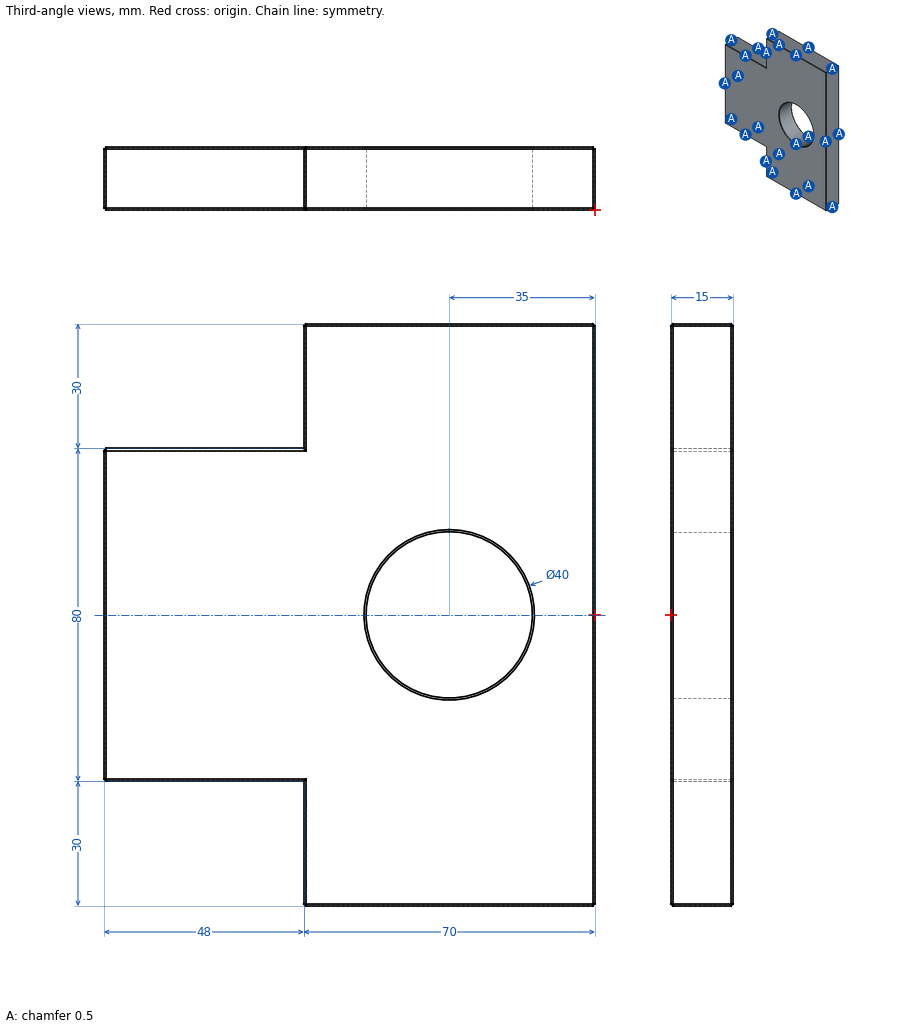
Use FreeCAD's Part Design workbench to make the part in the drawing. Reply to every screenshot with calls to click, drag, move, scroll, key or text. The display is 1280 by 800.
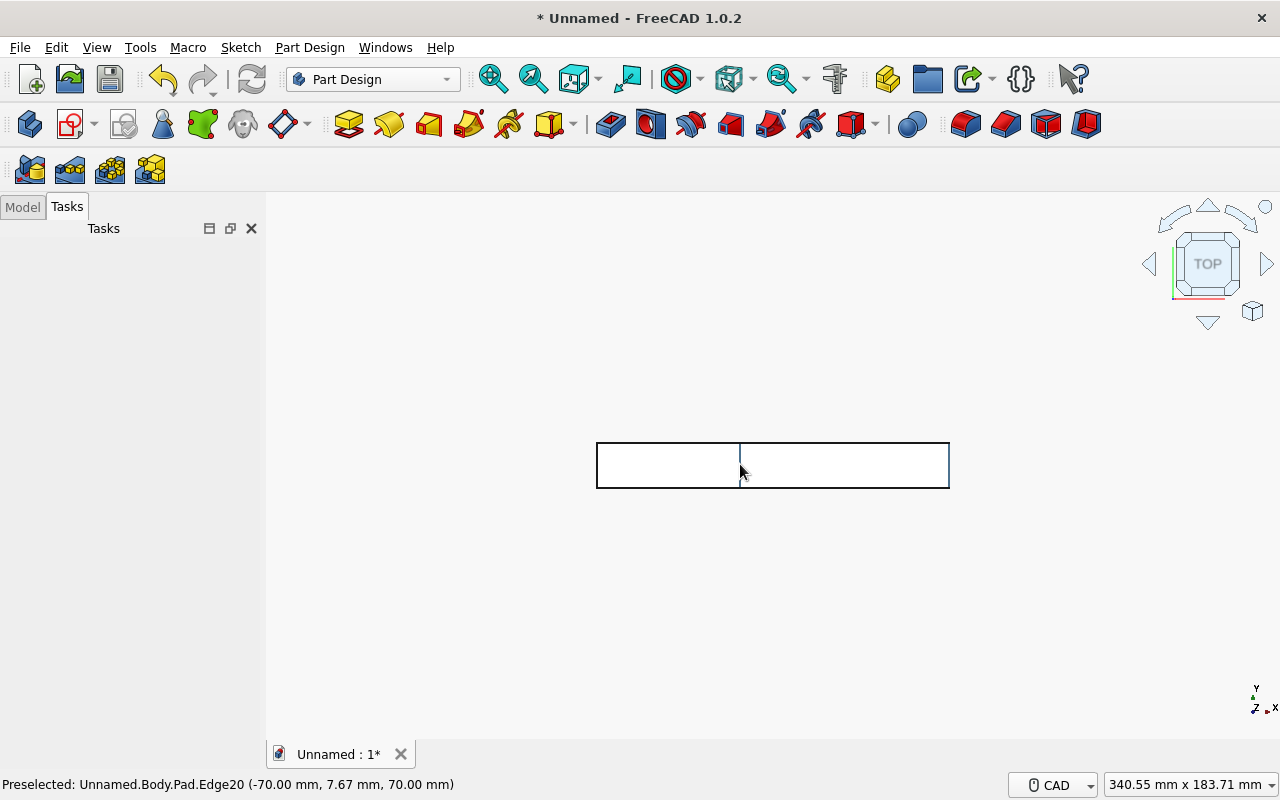
click(597, 464, ctrl)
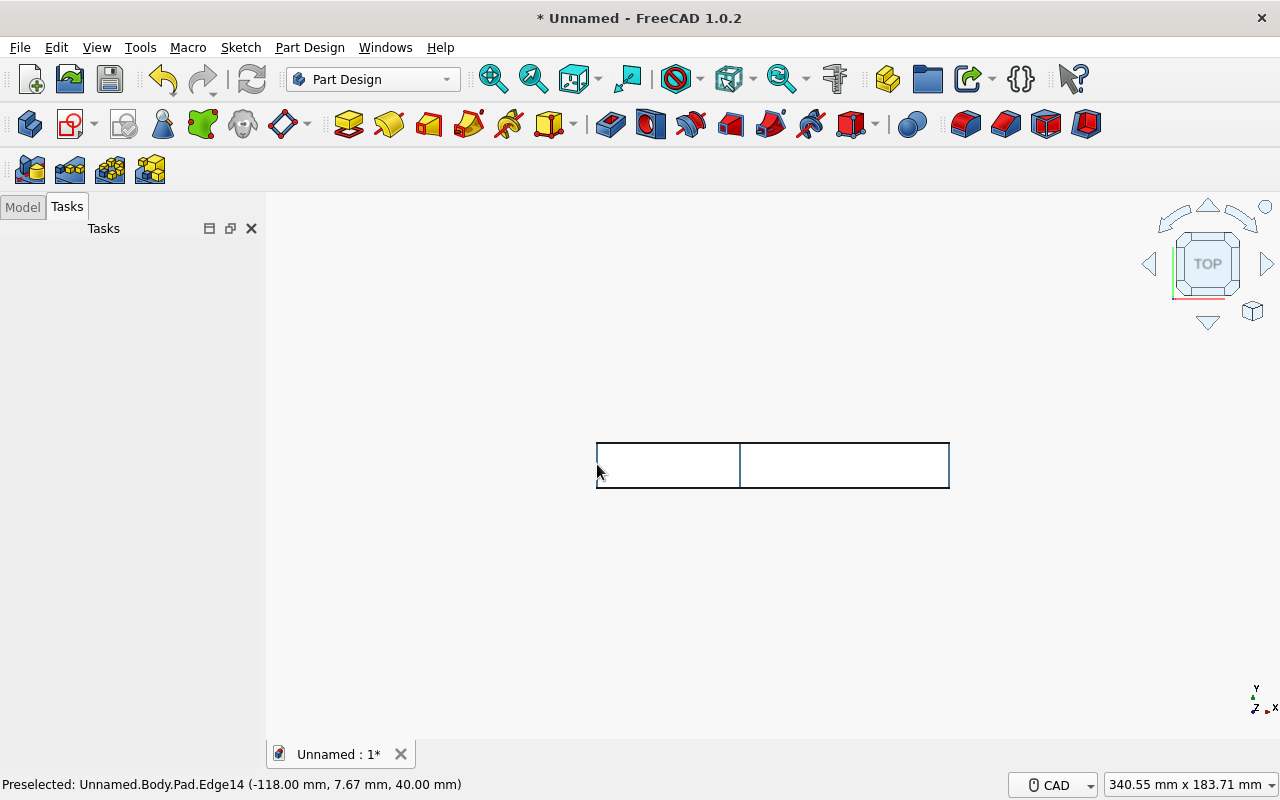
key(1)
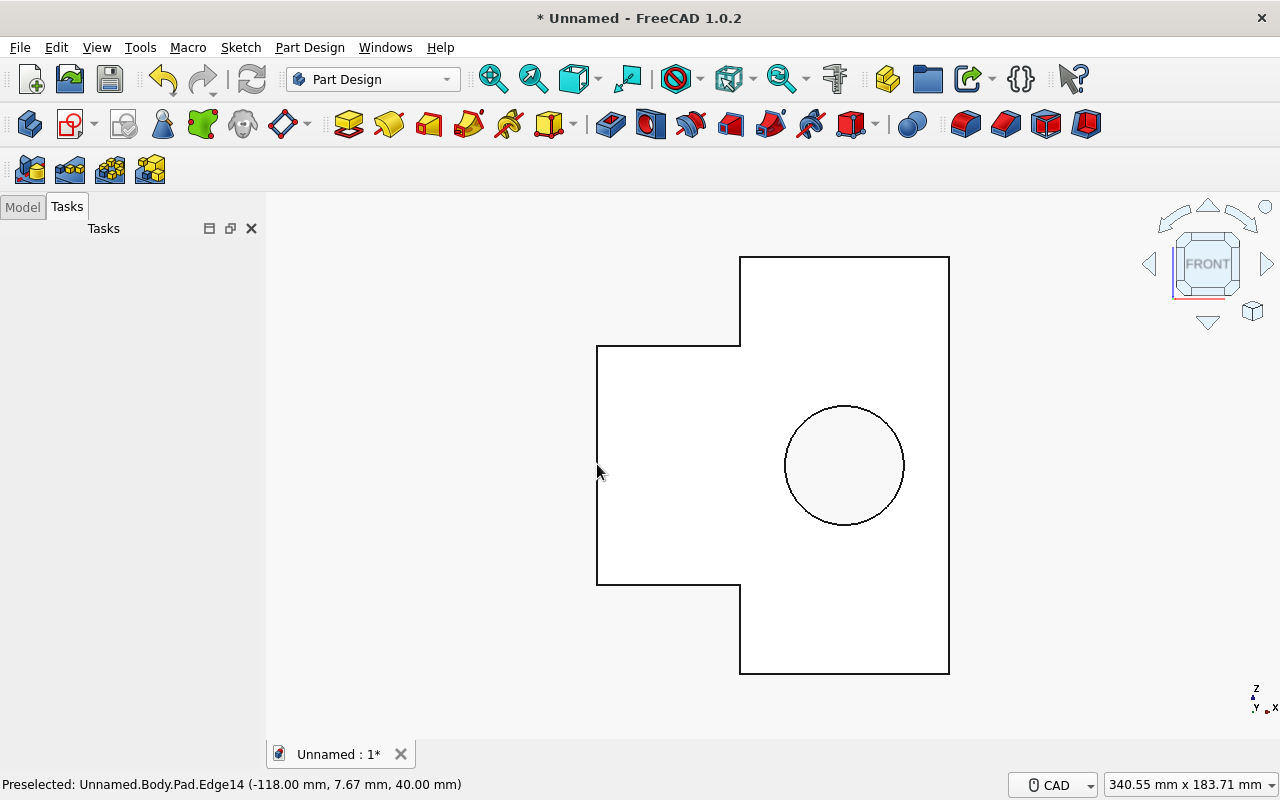
key(3)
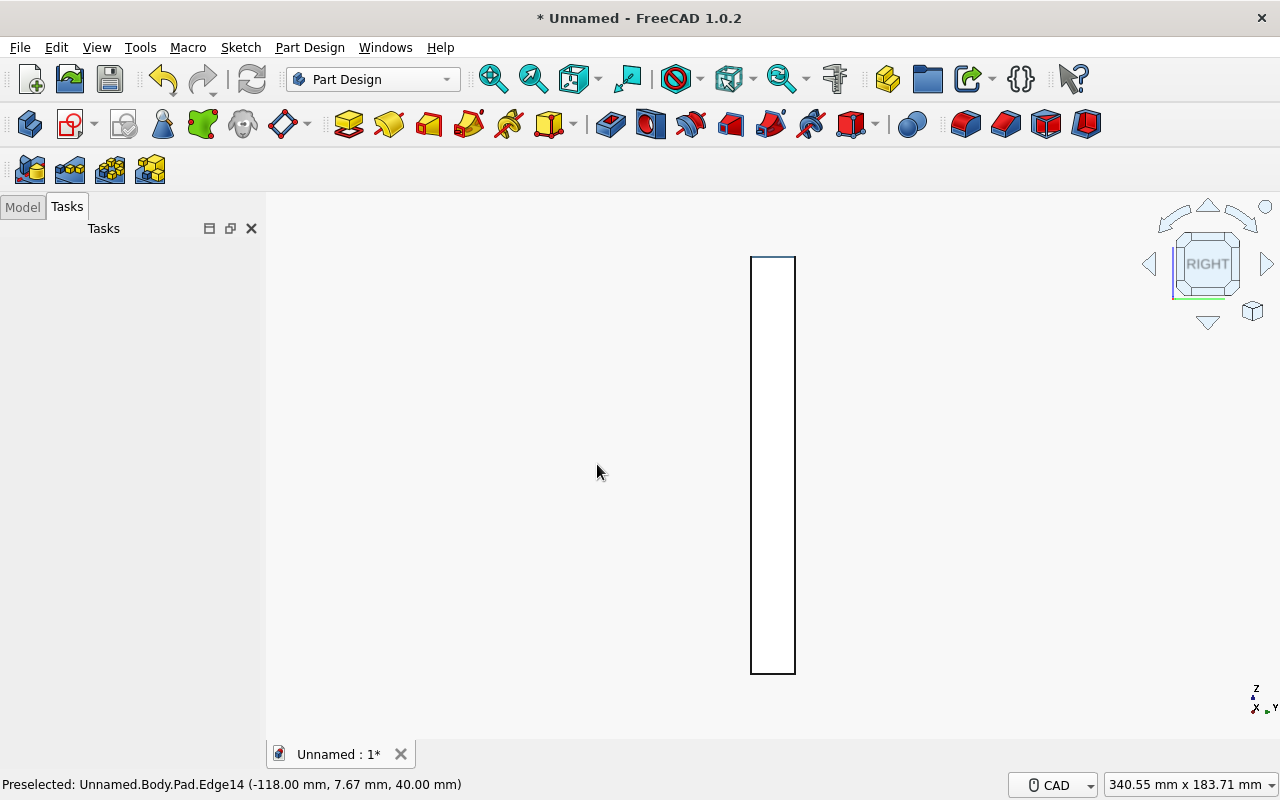
click(773, 673, ctrl)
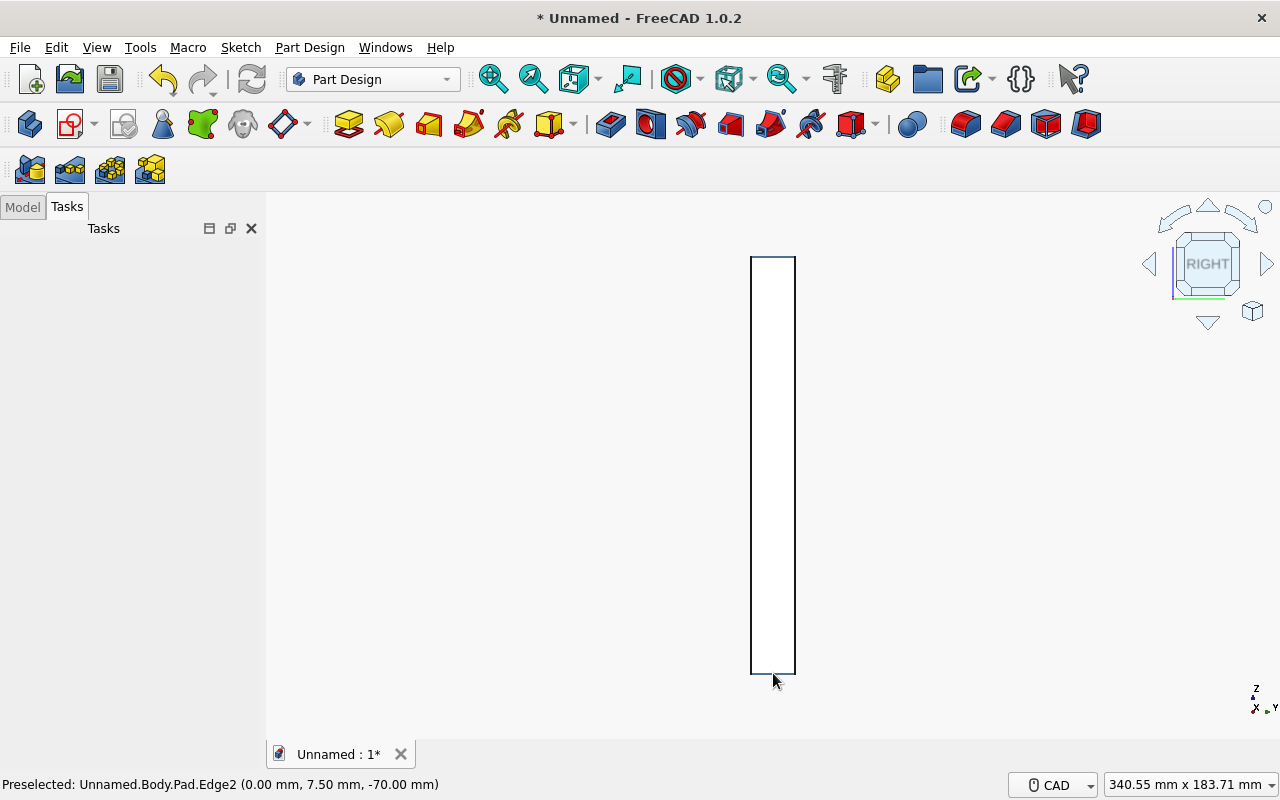
key(5)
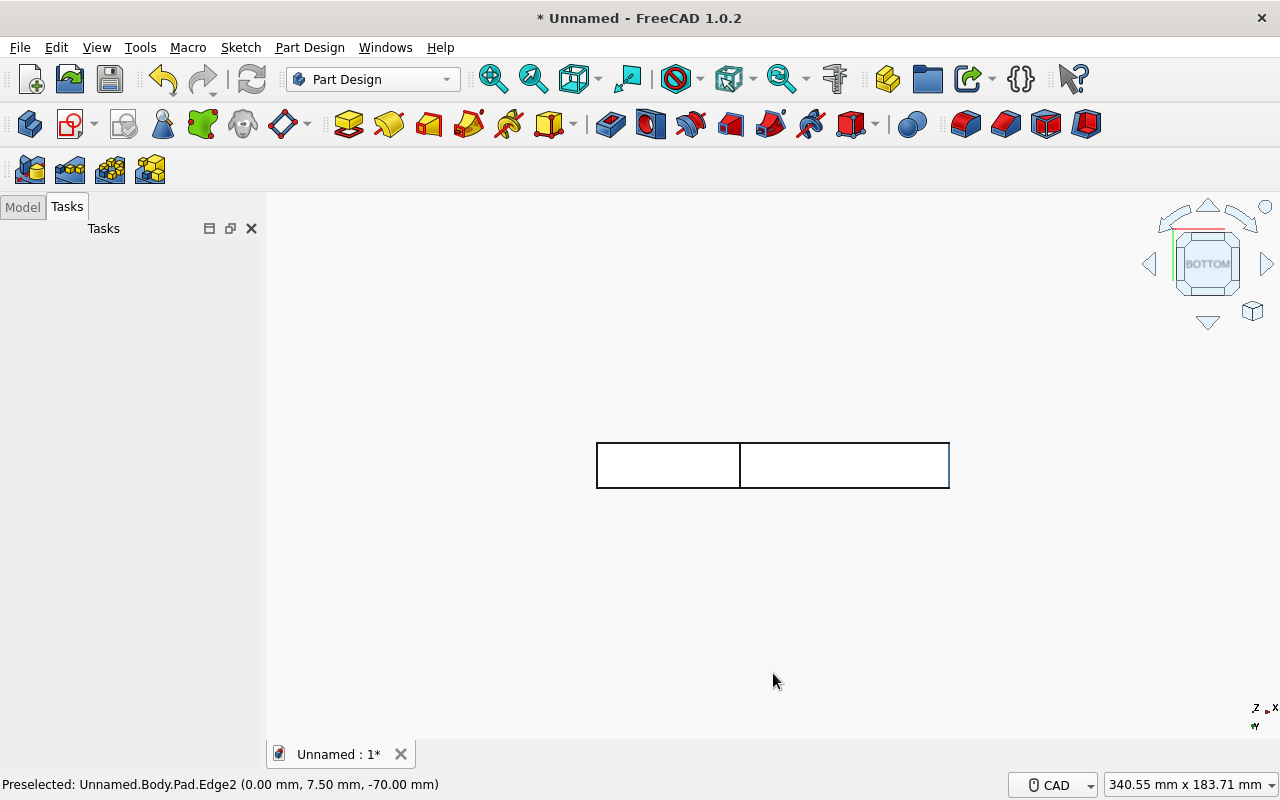
click(494, 80)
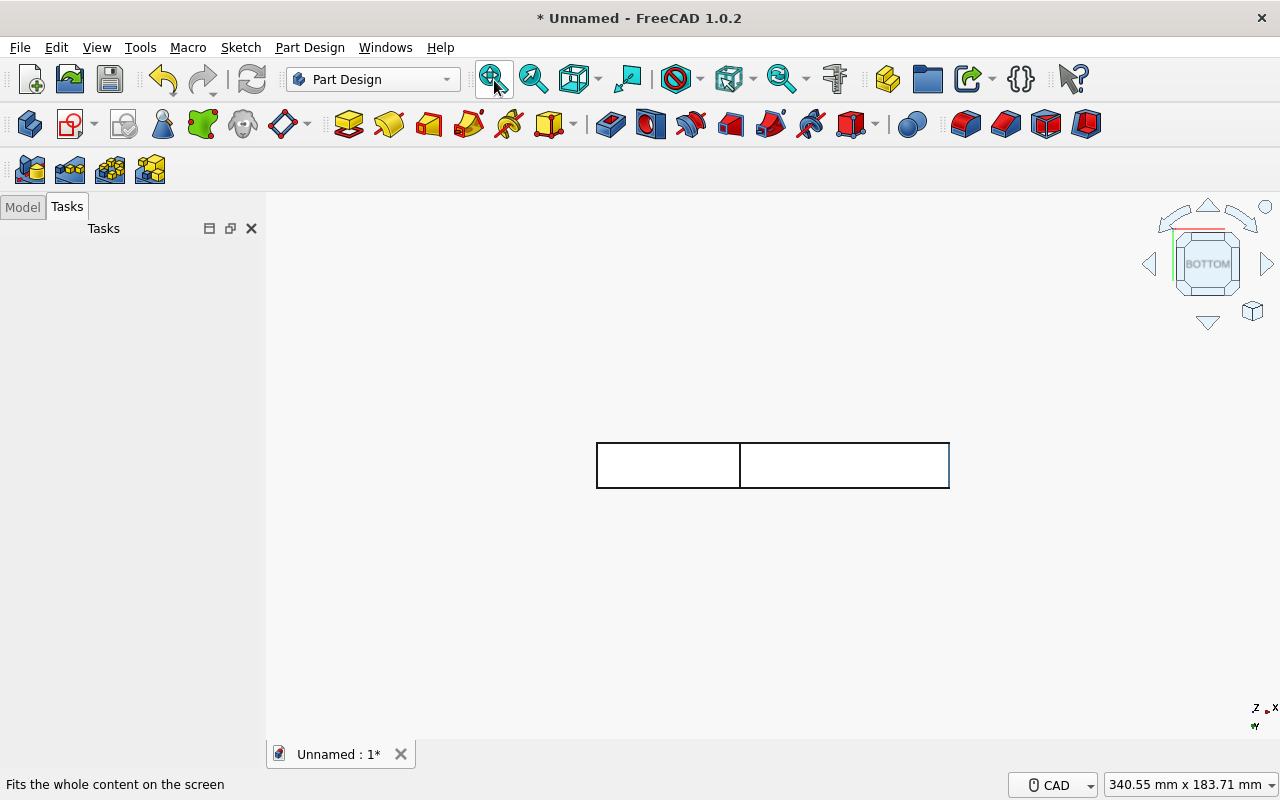
click(597, 464, ctrl)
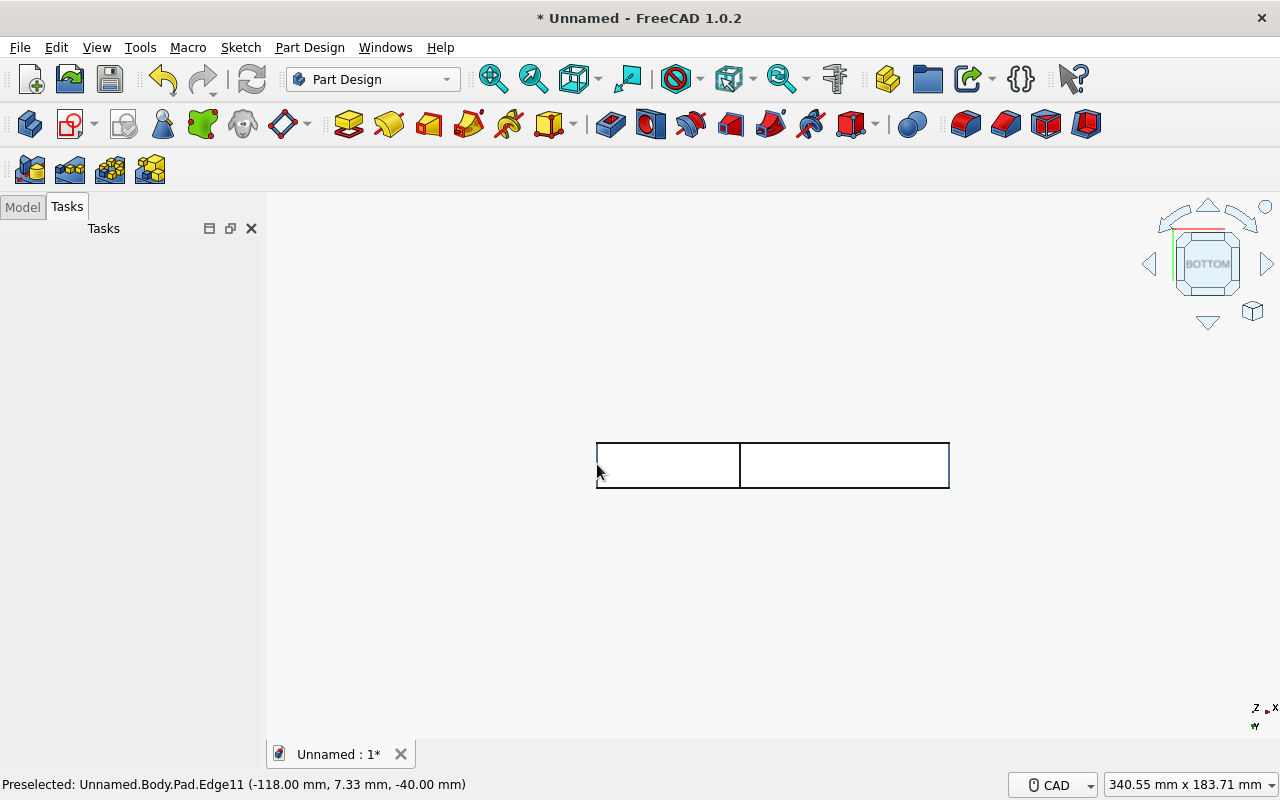
click(740, 464, ctrl)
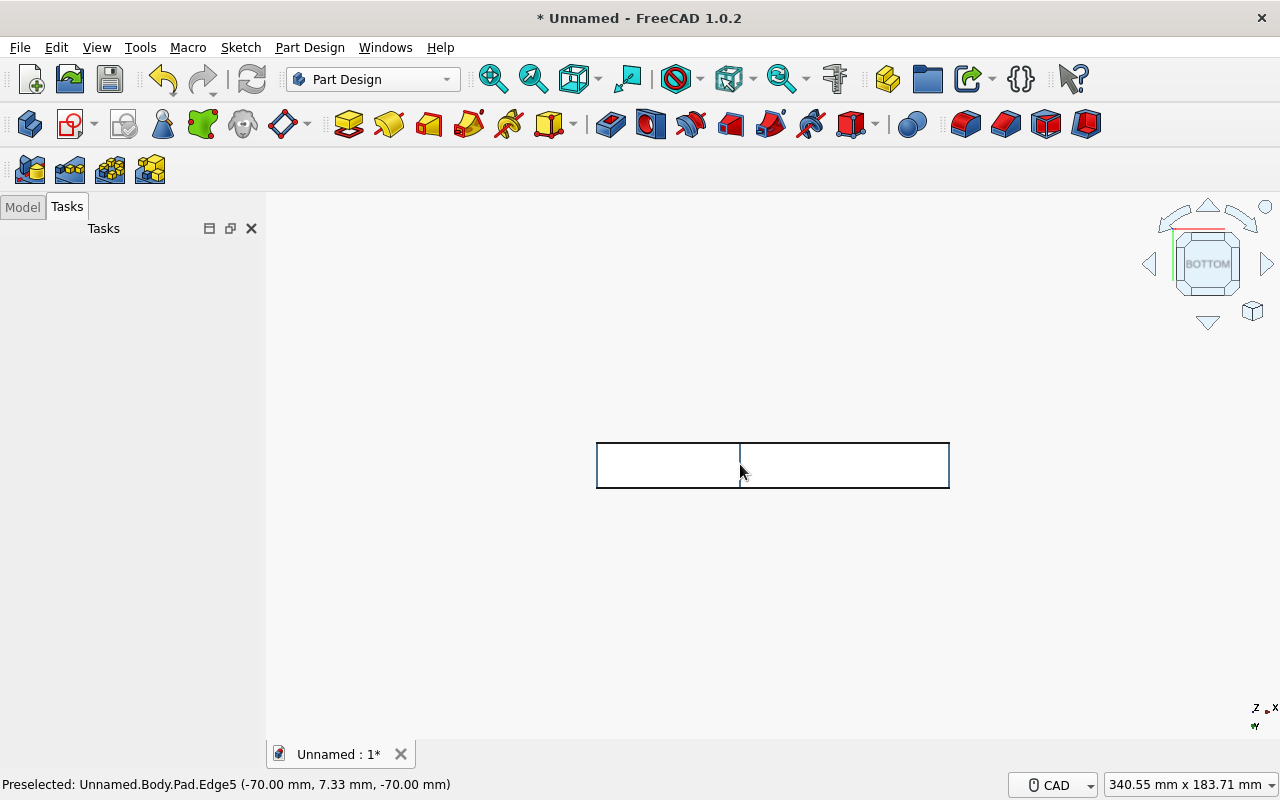
key(4)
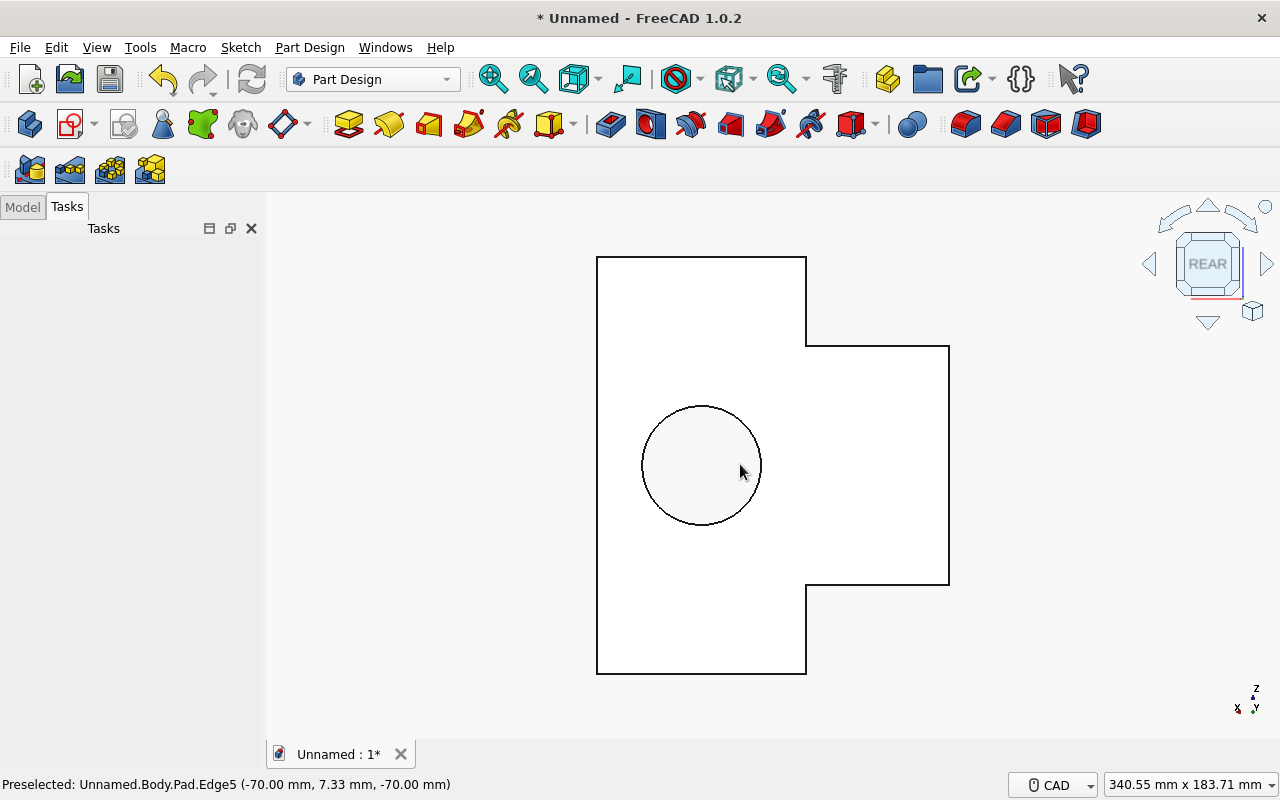
click(873, 465, ctrl)